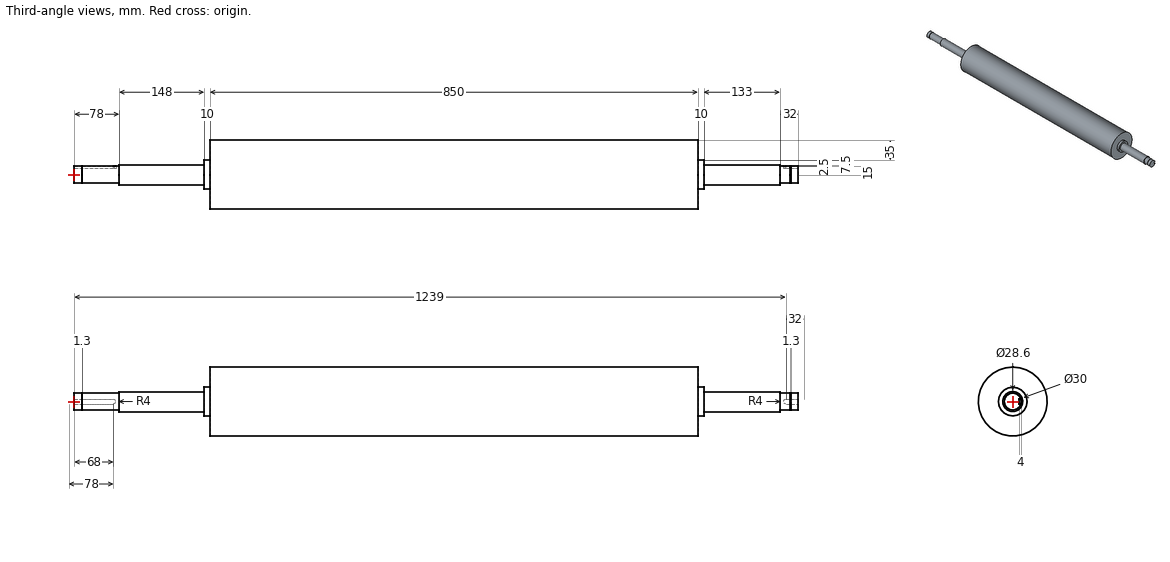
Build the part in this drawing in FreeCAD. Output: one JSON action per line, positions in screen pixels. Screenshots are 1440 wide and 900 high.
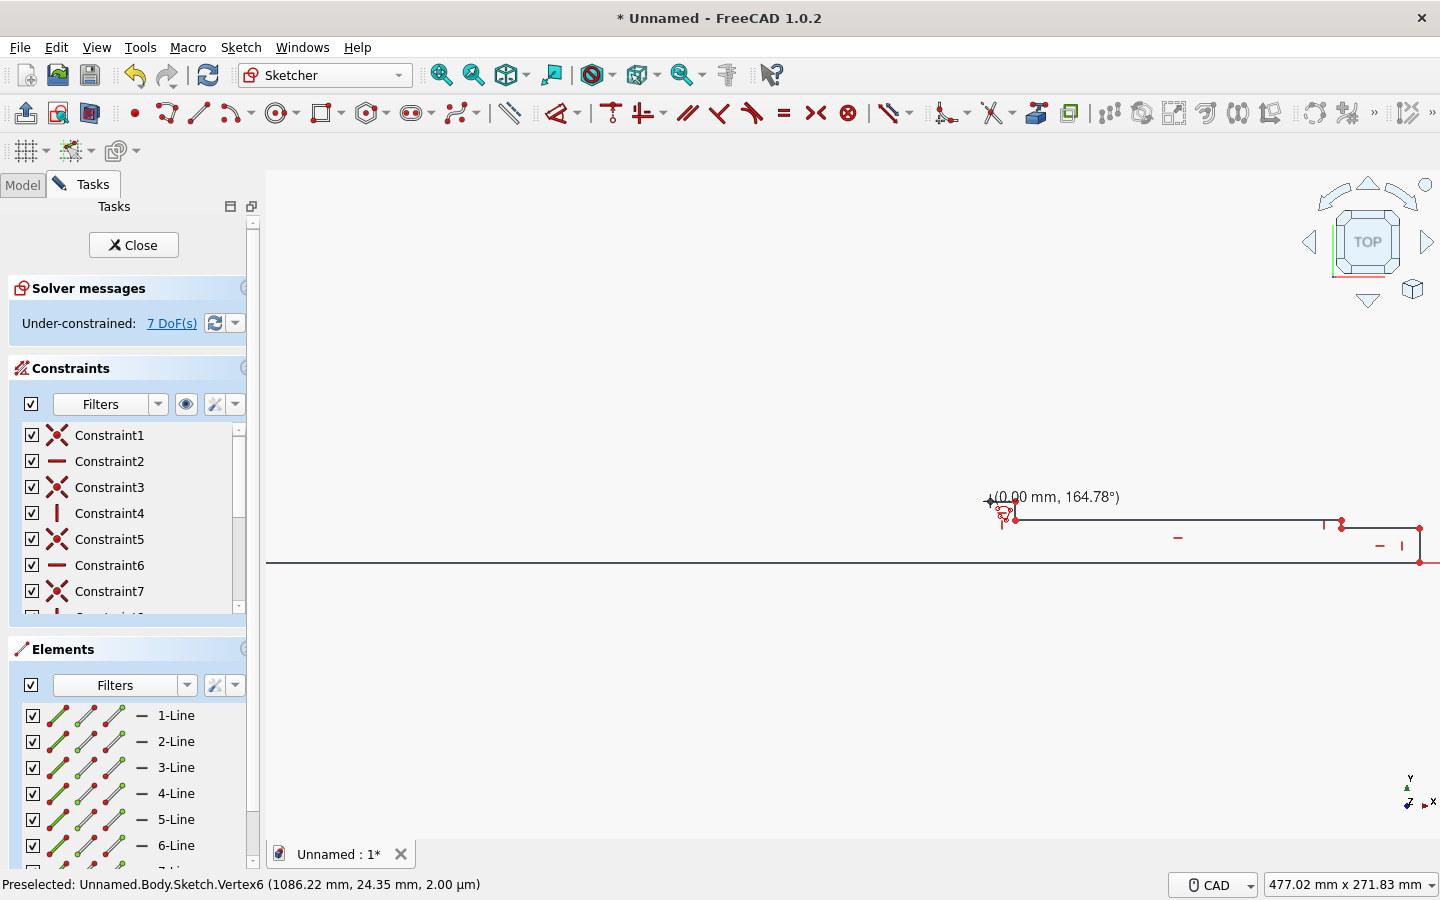
{"action": "scroll", "coordinate": [1016, 508], "scroll_direction": "down", "scroll_amount": 8}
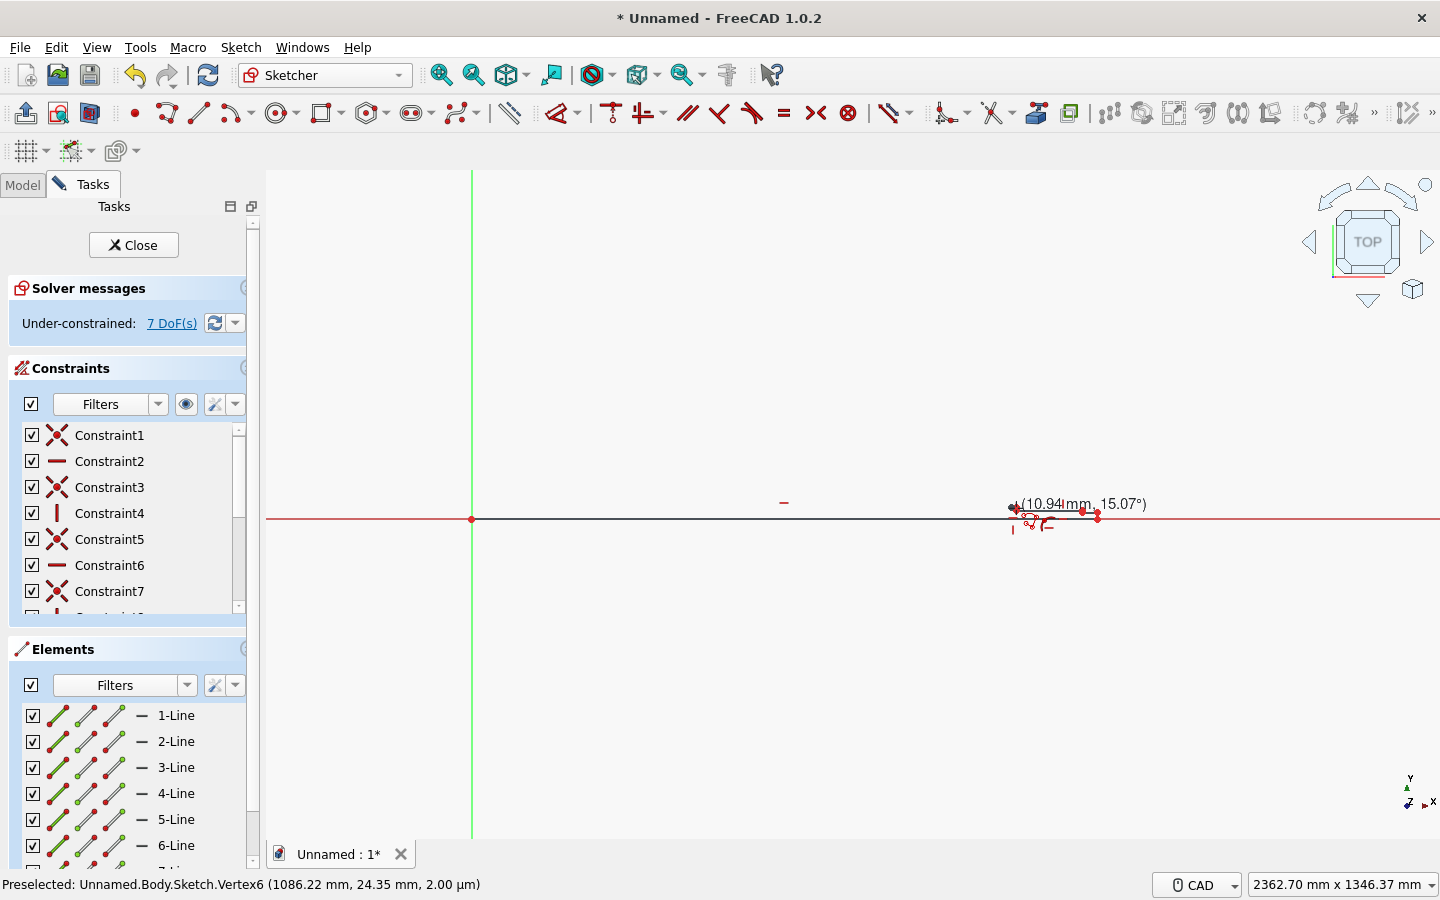
{"action": "left_click", "coordinate": [1011, 490]}
{"action": "left_click", "coordinate": [589, 490]}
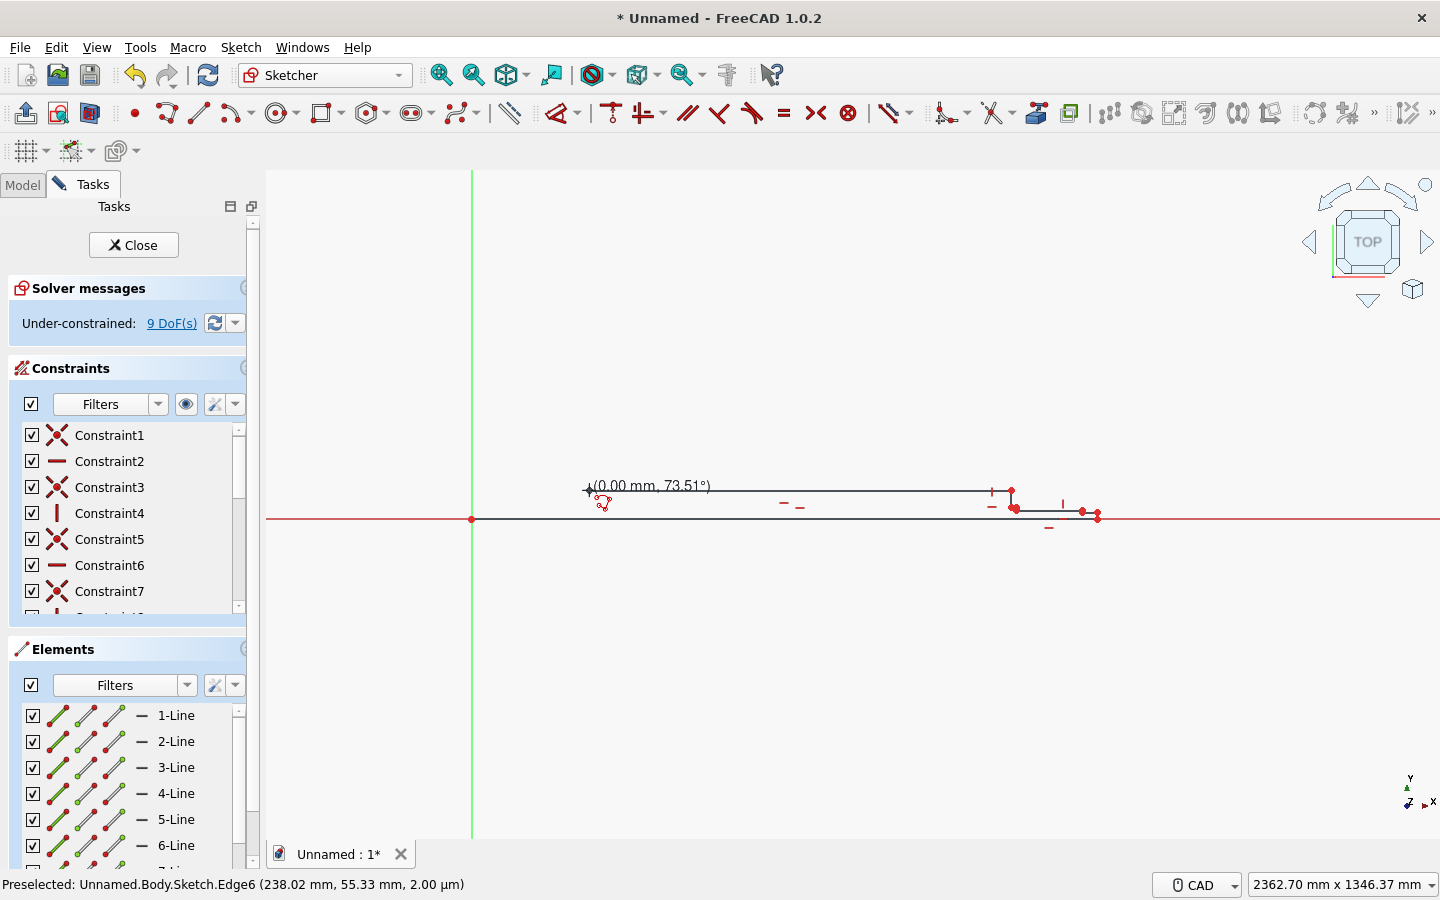
{"action": "scroll", "coordinate": [589, 507], "scroll_direction": "up", "scroll_amount": 2}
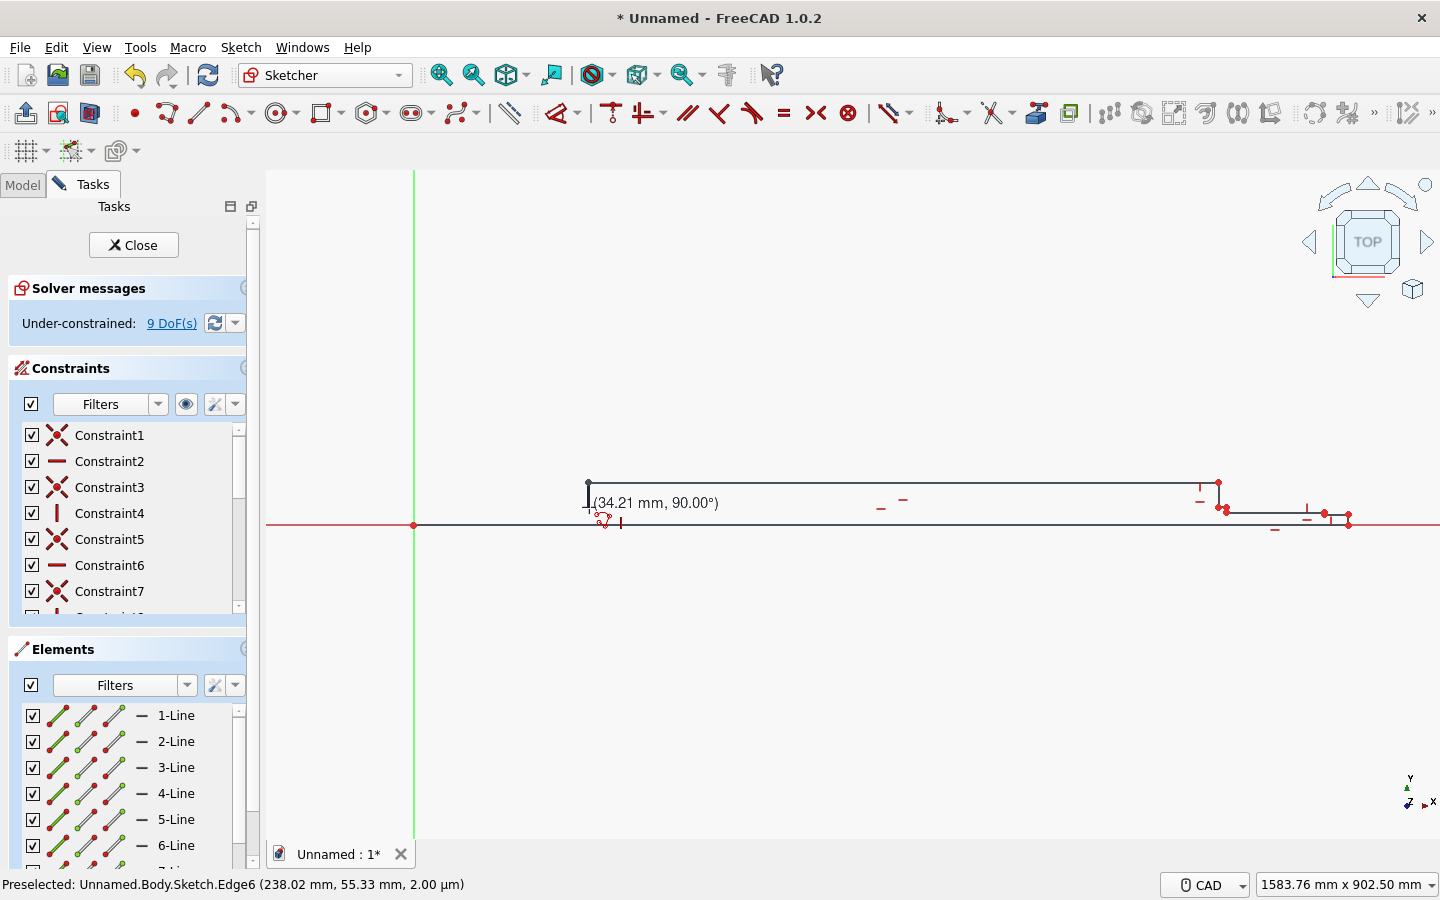
{"action": "left_click", "coordinate": [589, 507]}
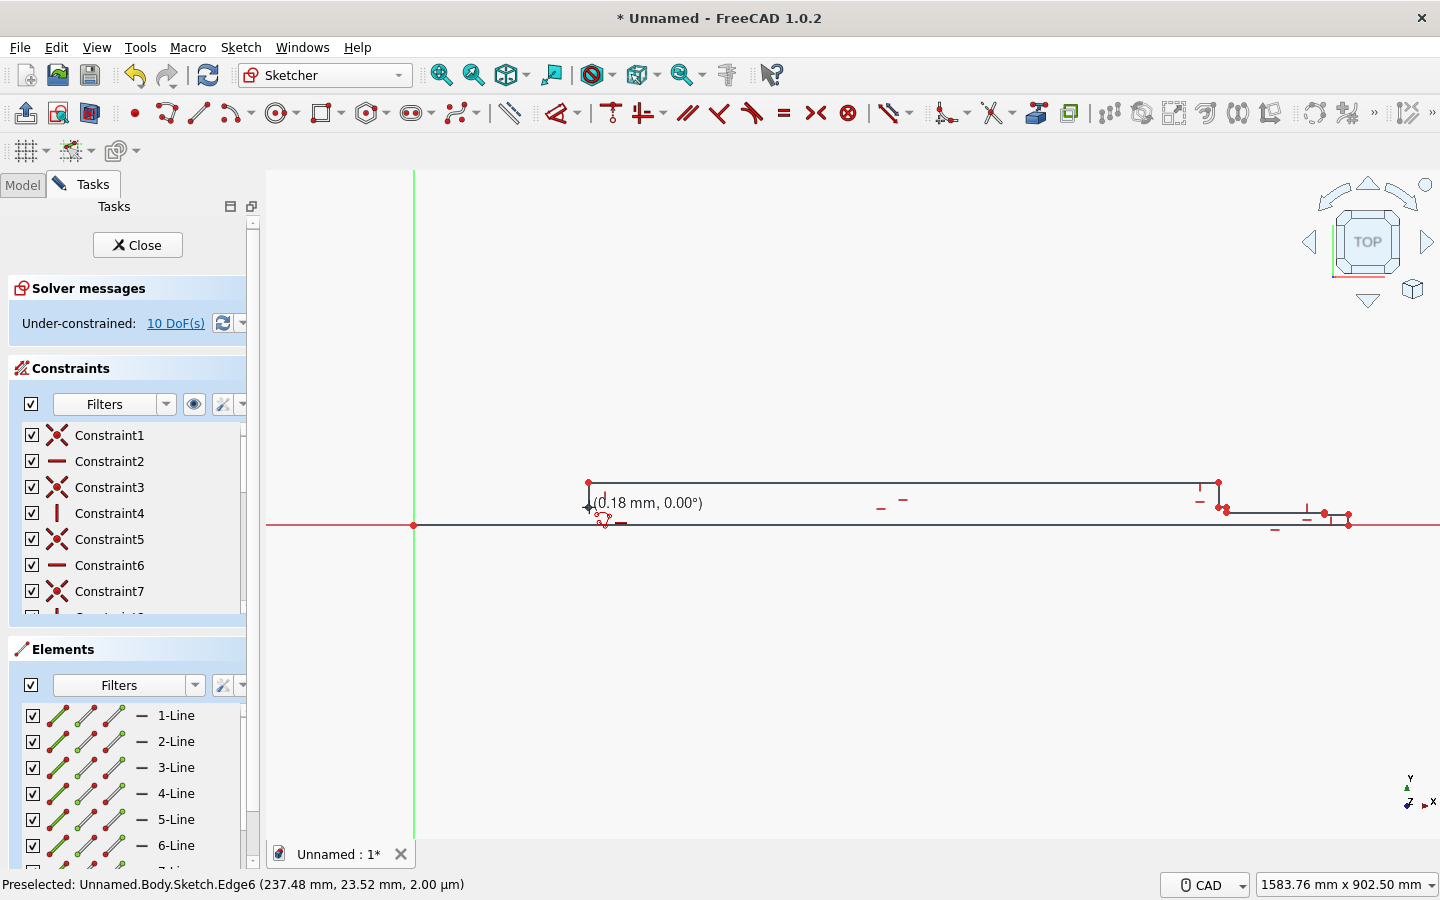
{"action": "scroll", "coordinate": [581, 507], "scroll_direction": "up", "scroll_amount": 4}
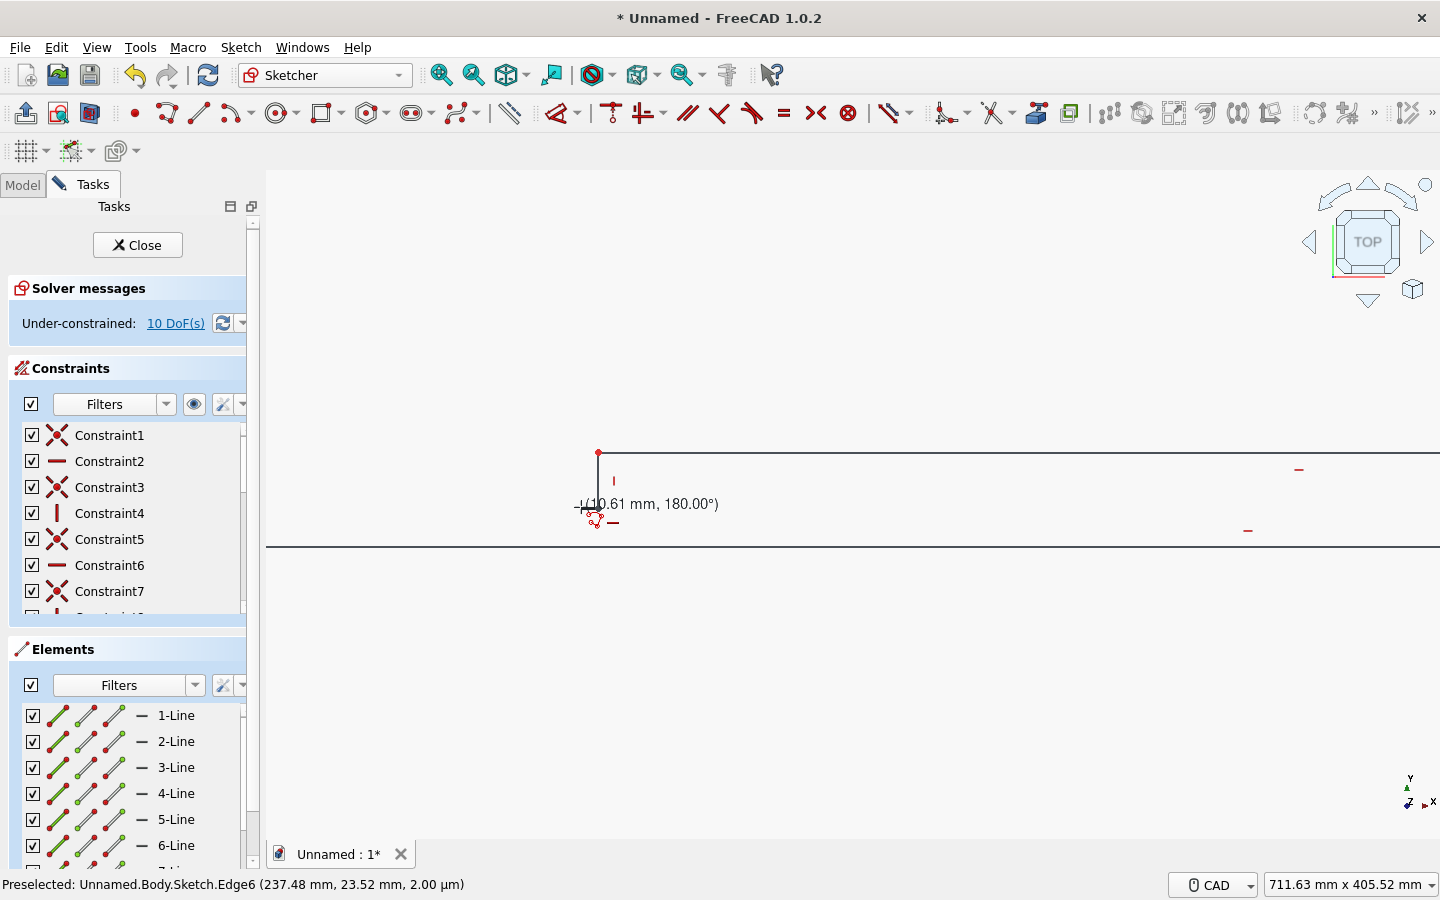
{"action": "left_click", "coordinate": [582, 506]}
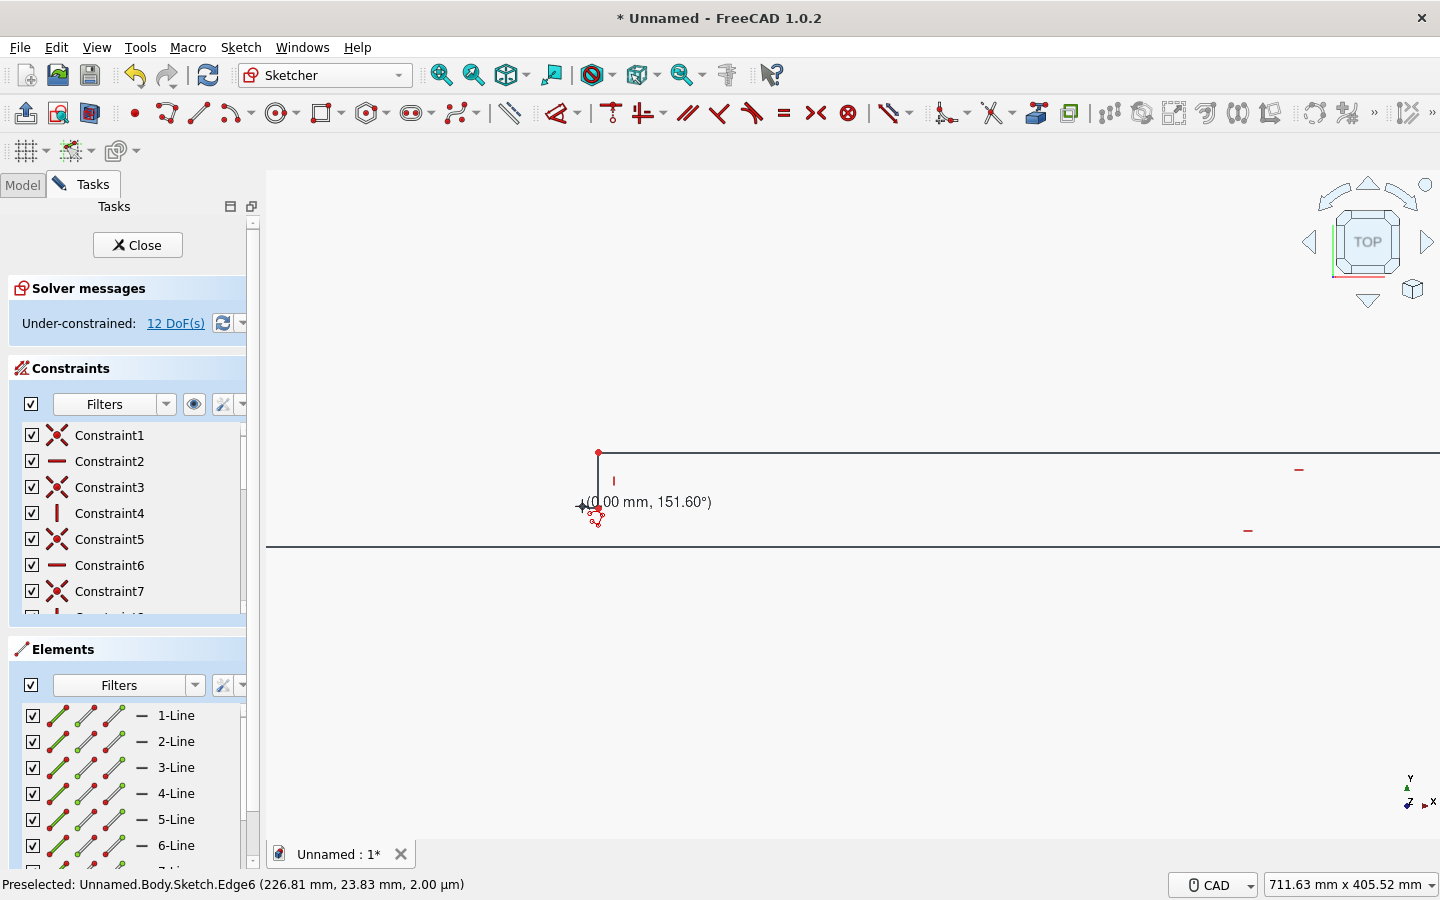
{"action": "scroll", "coordinate": [582, 518], "scroll_direction": "up", "scroll_amount": 2}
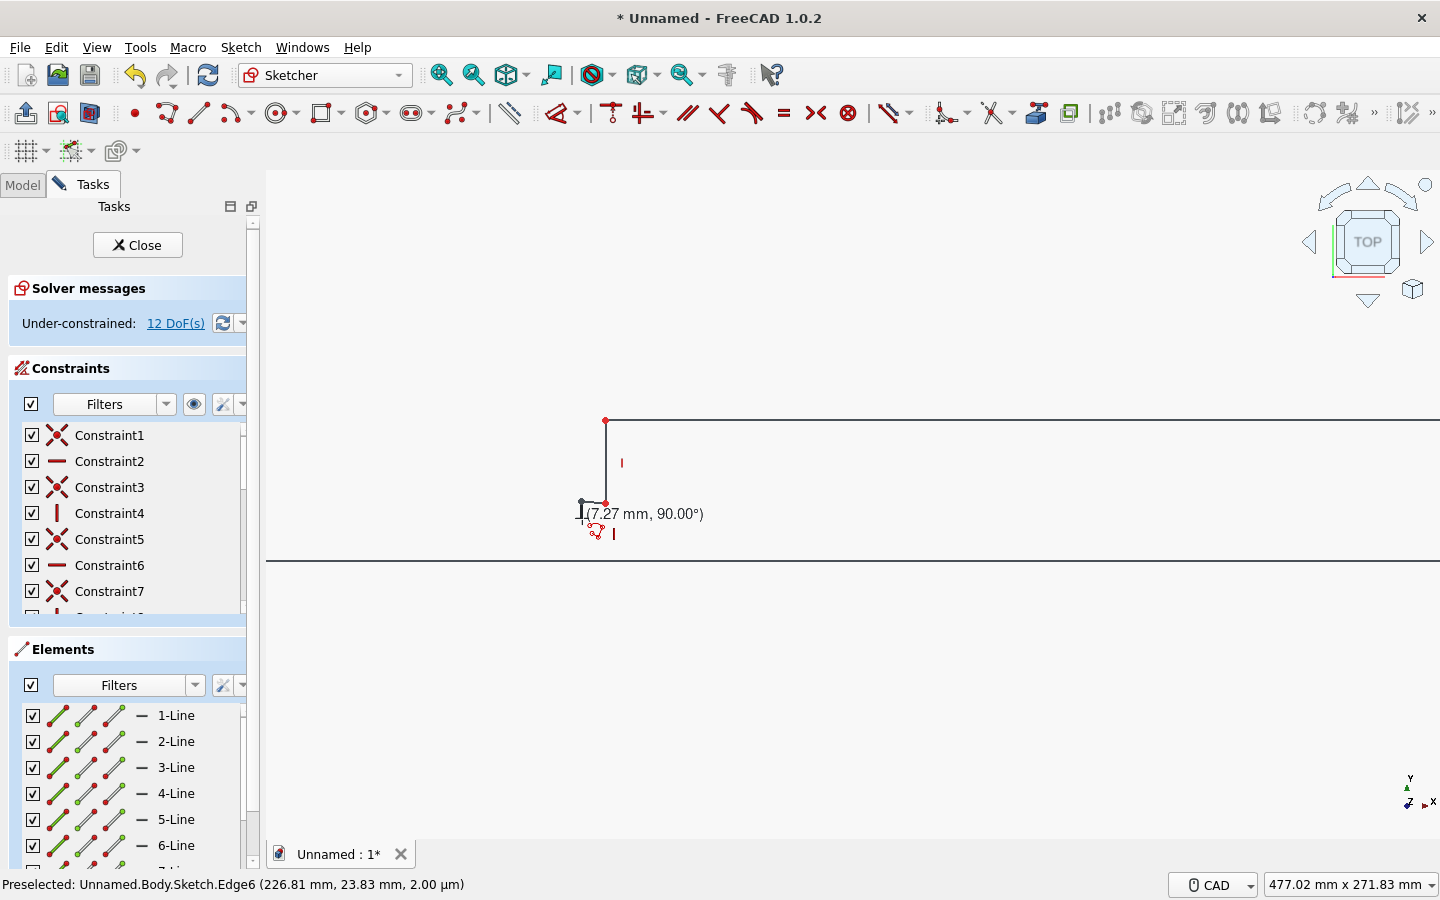
{"action": "left_click", "coordinate": [582, 518]}